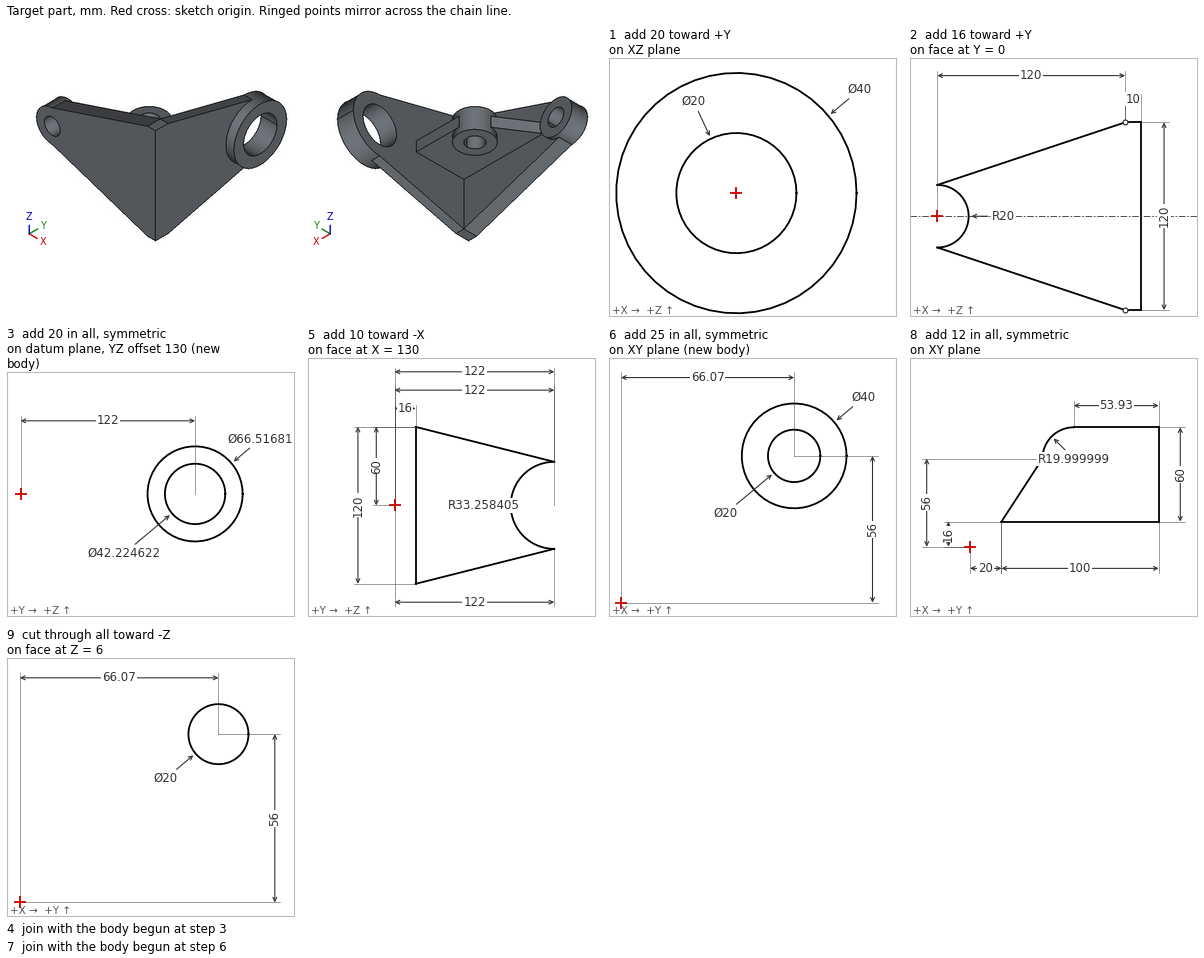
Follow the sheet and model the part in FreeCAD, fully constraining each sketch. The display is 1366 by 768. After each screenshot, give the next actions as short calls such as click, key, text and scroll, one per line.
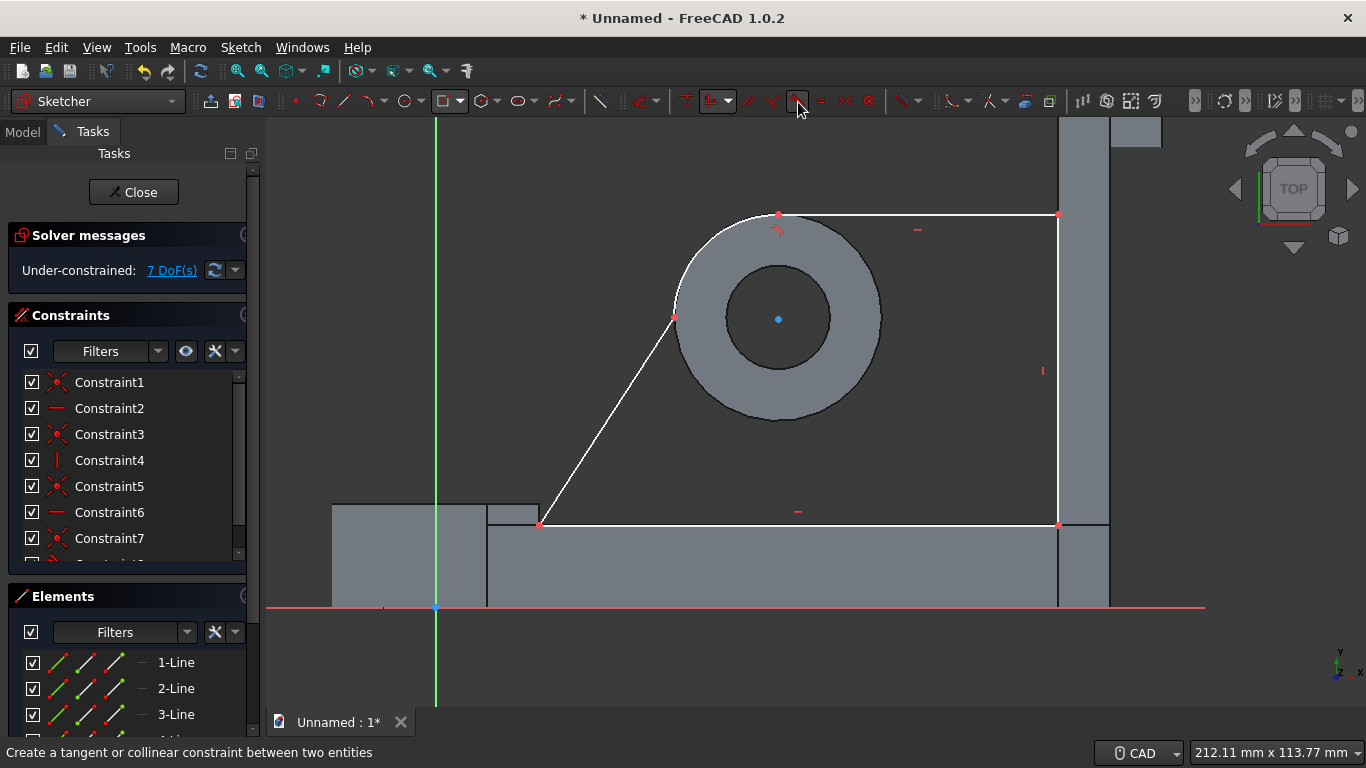
click(640, 102)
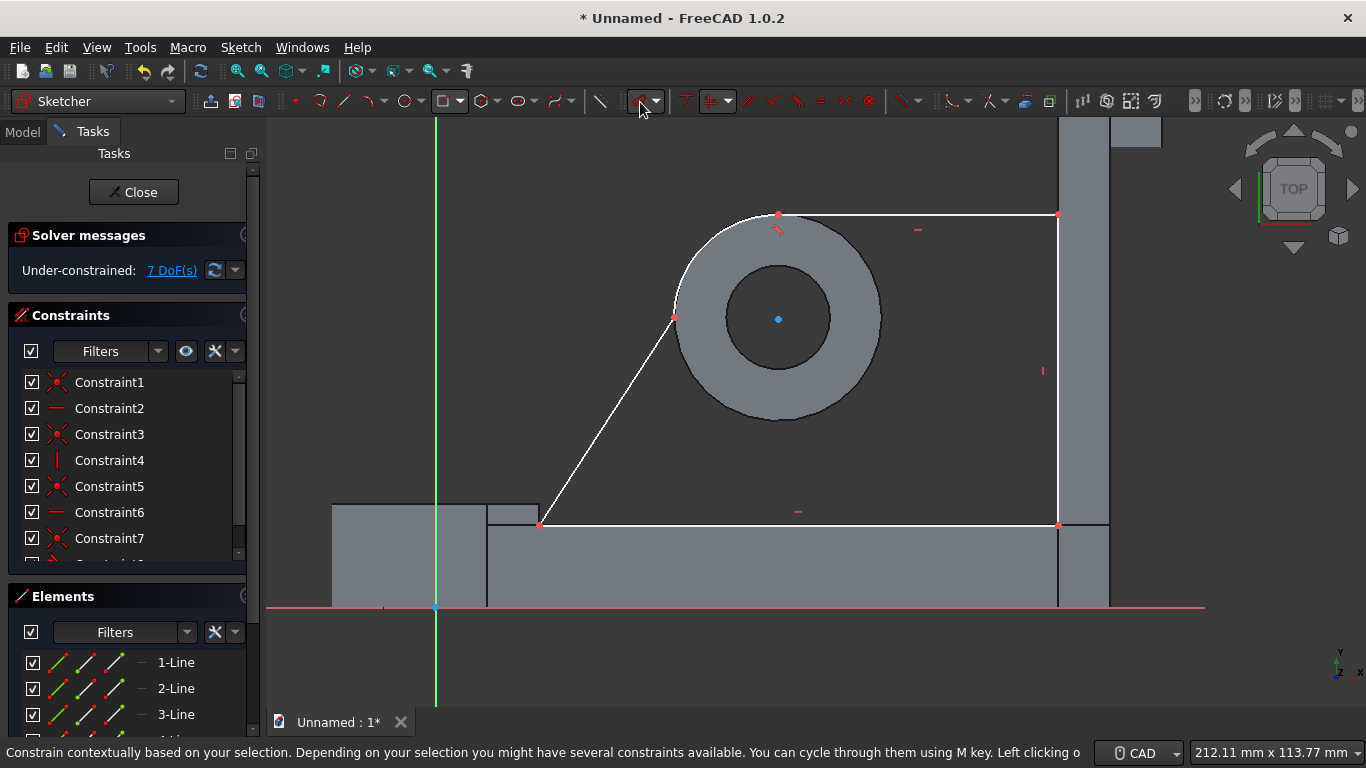
click(731, 226)
click(717, 197)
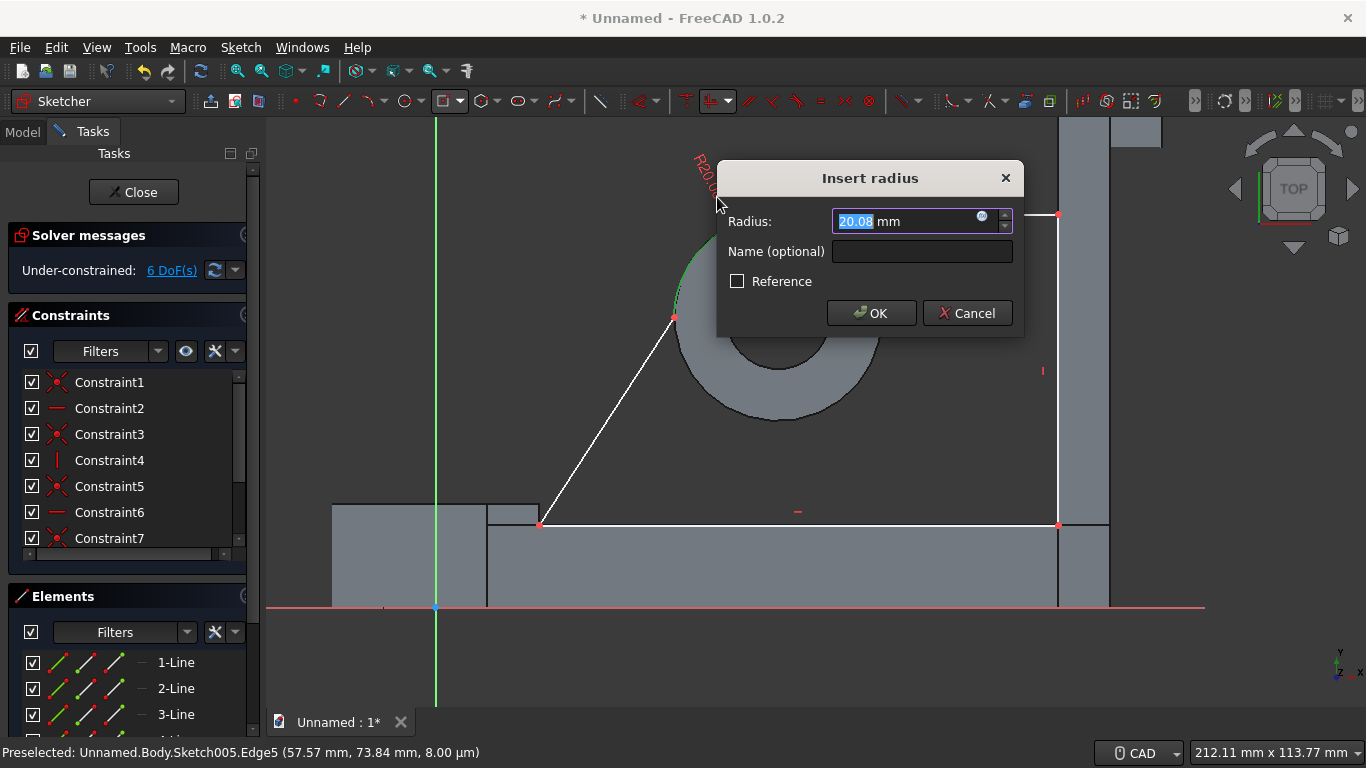
text(19.999999)
key(Return)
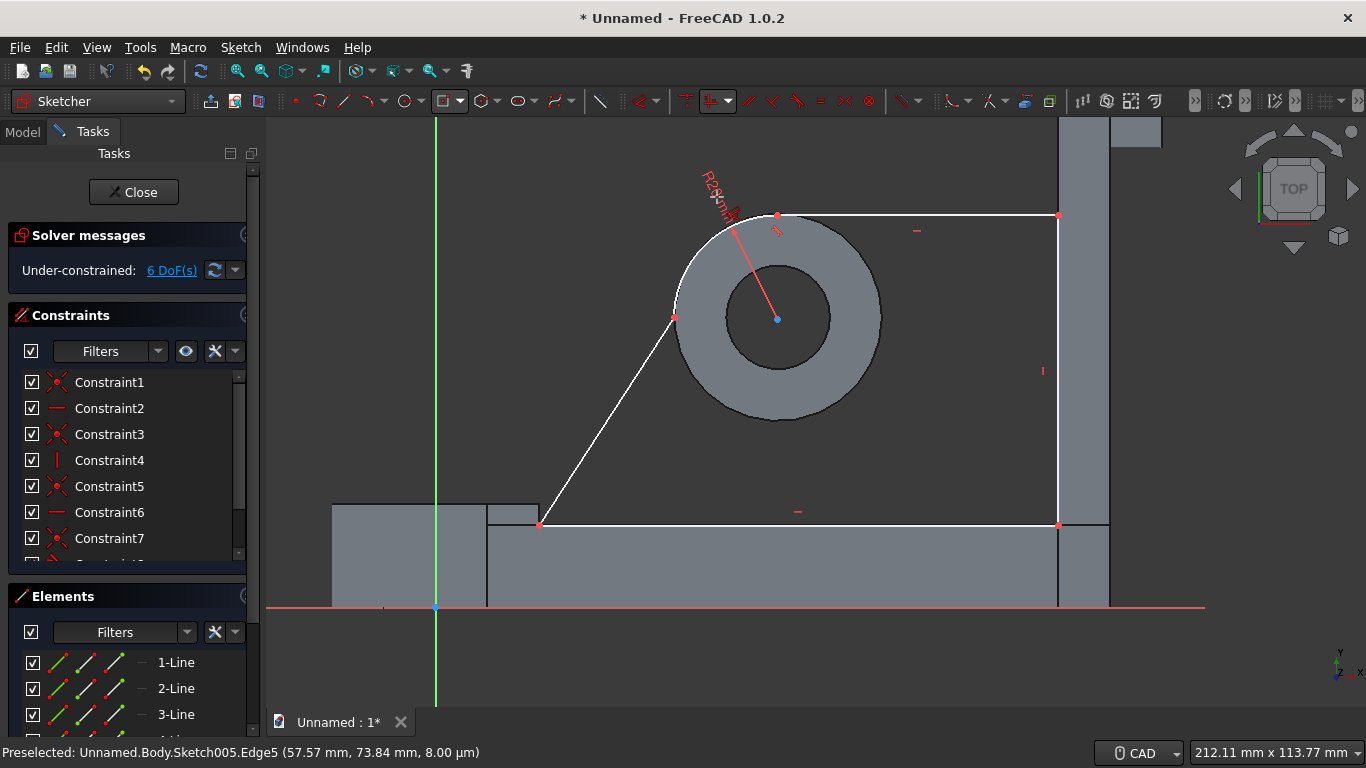
click(1058, 433)
click(1092, 371)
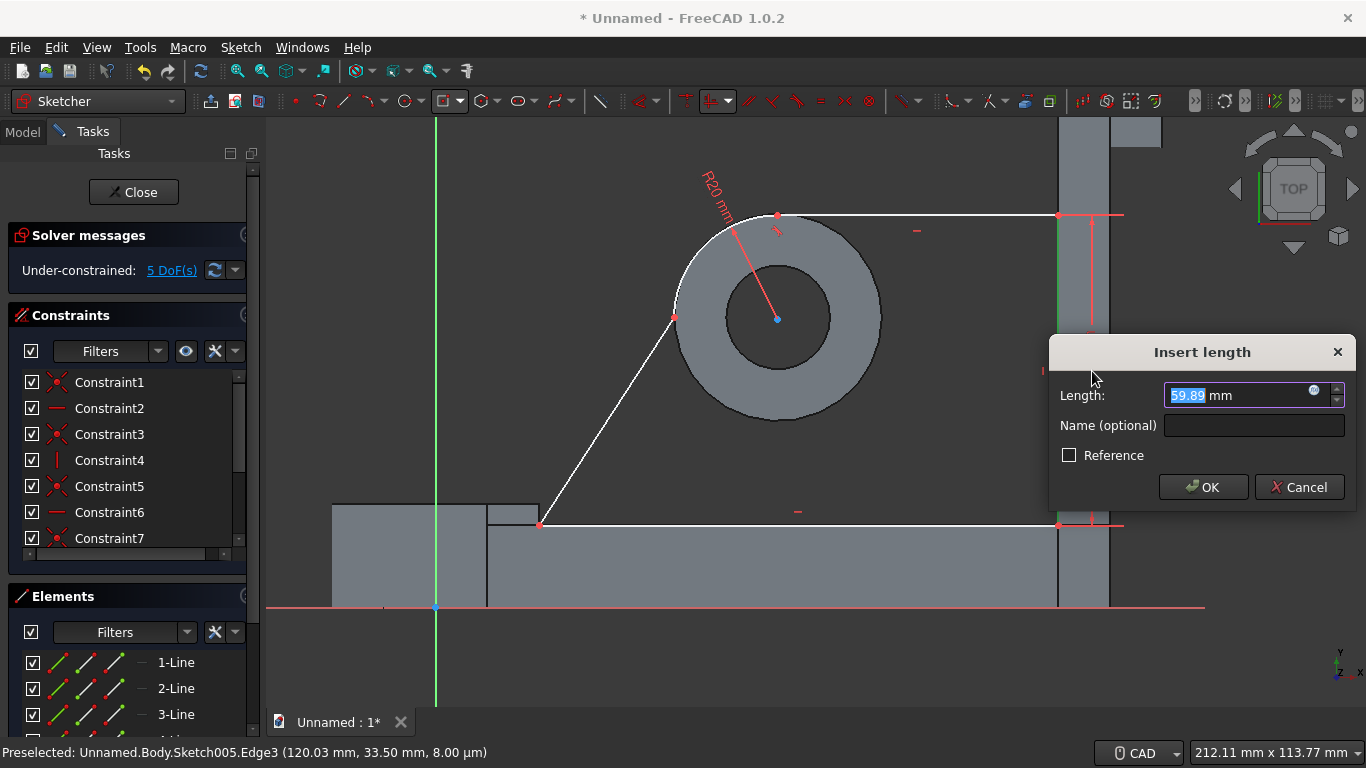
text(60)
key(Return)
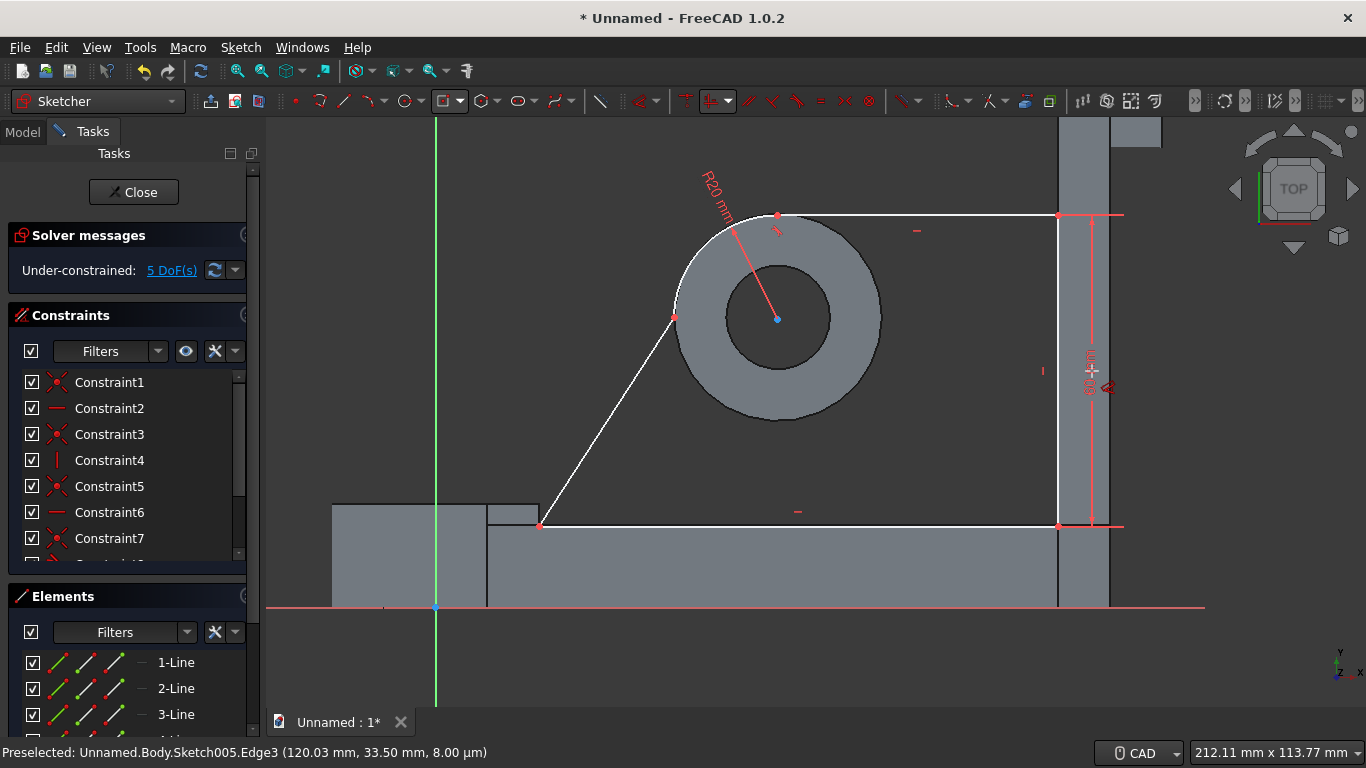
click(695, 527)
click(799, 561)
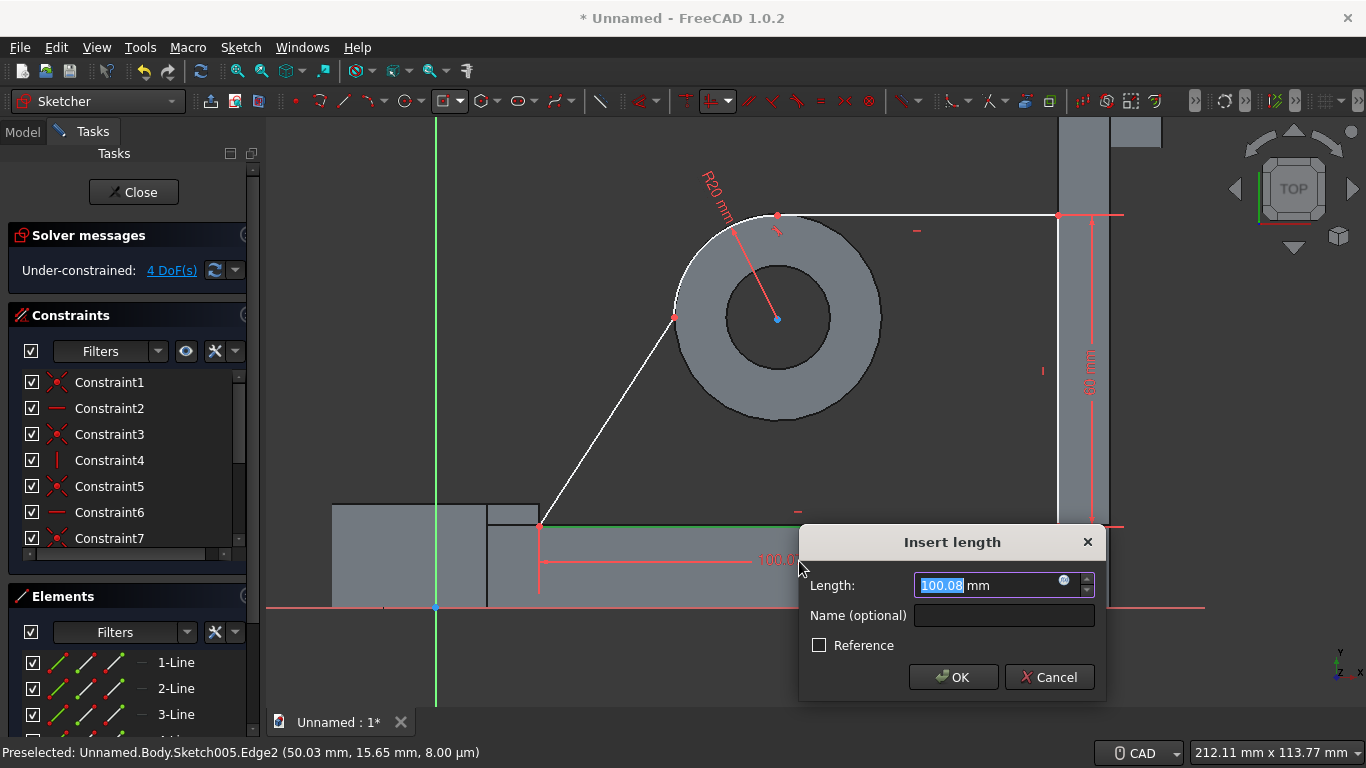
text(100)
key(Return)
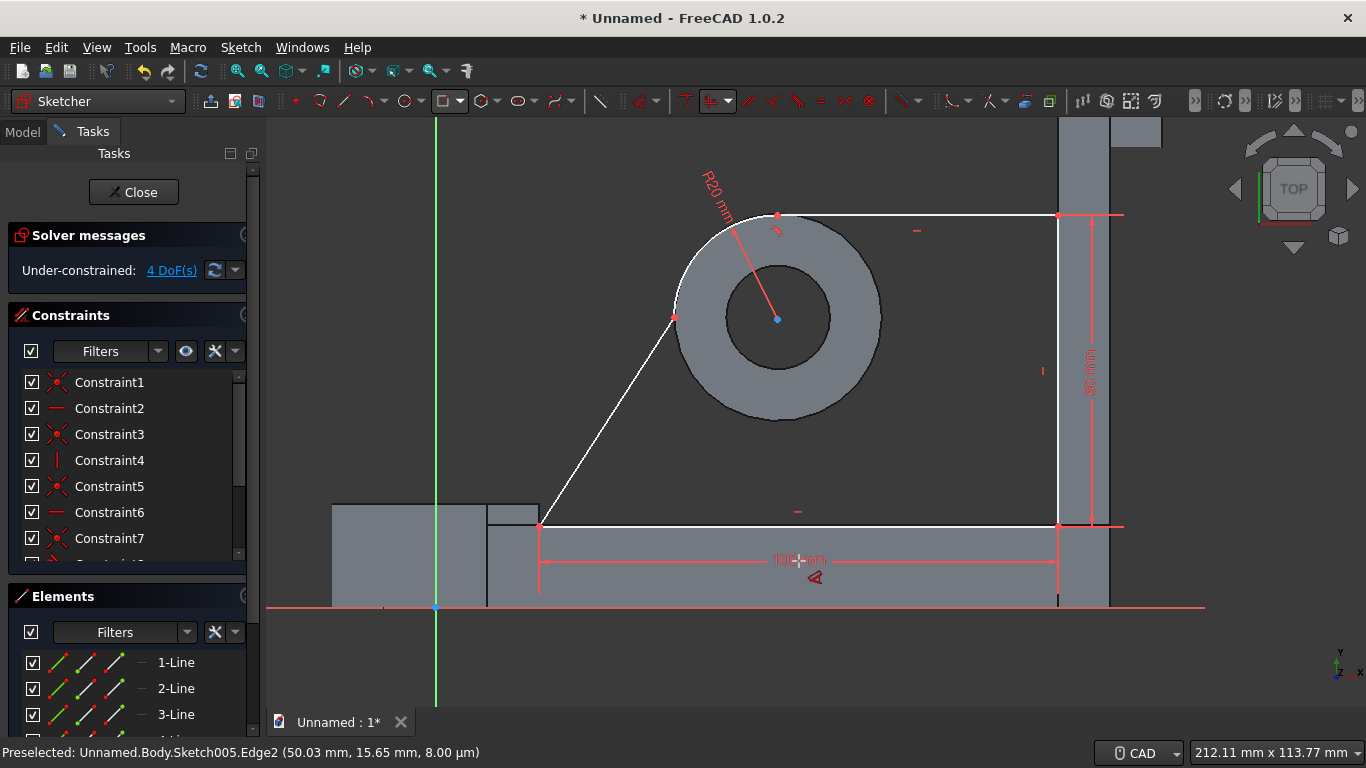
click(674, 318)
click(402, 463)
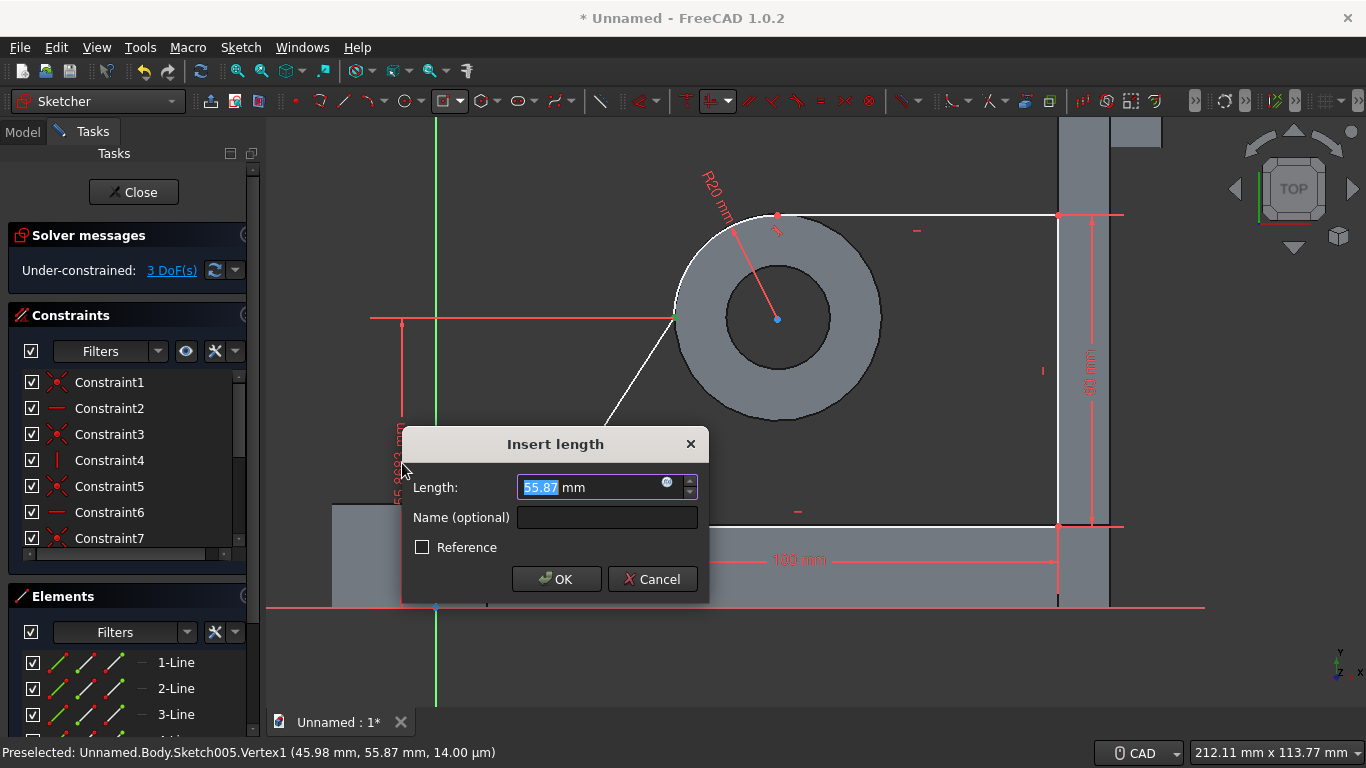
text(56)
key(Return)